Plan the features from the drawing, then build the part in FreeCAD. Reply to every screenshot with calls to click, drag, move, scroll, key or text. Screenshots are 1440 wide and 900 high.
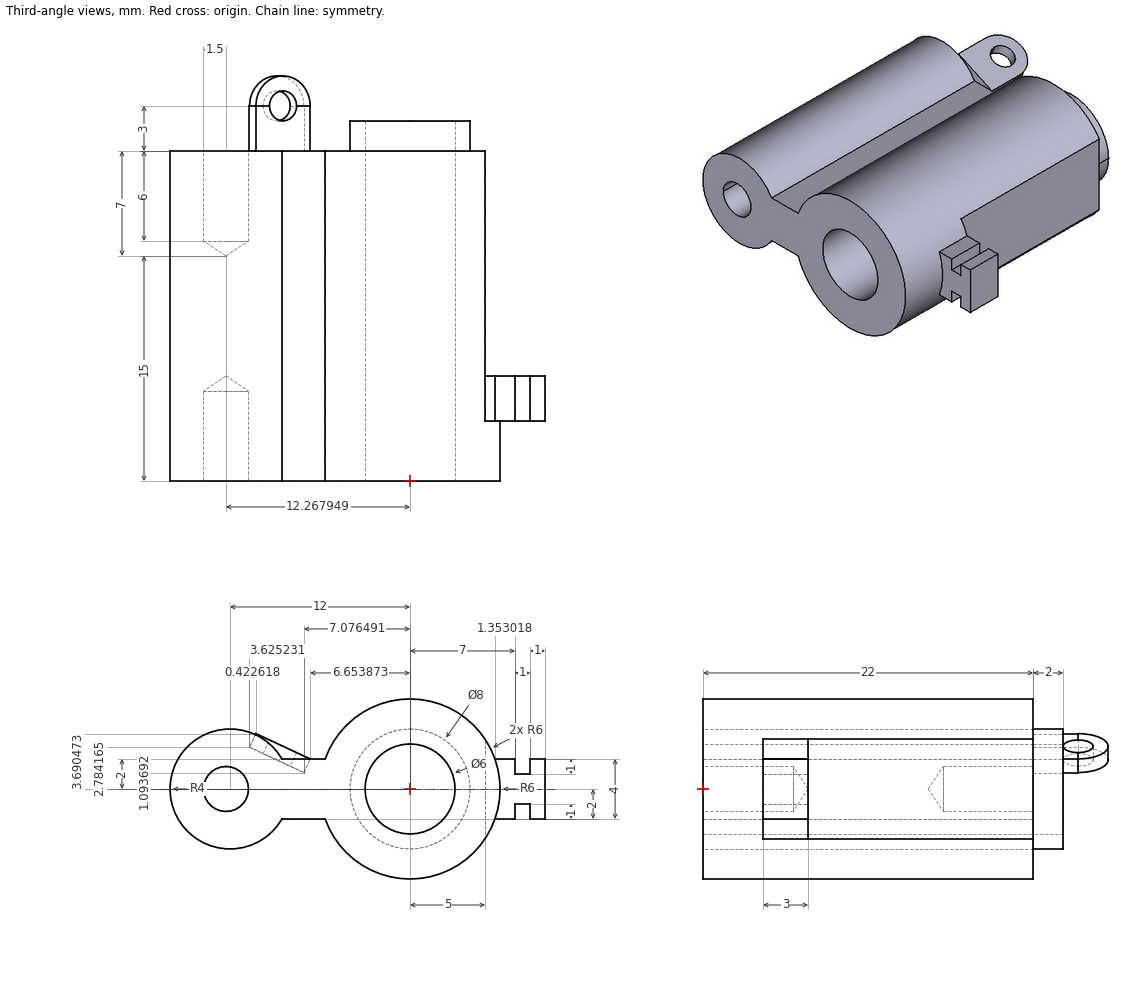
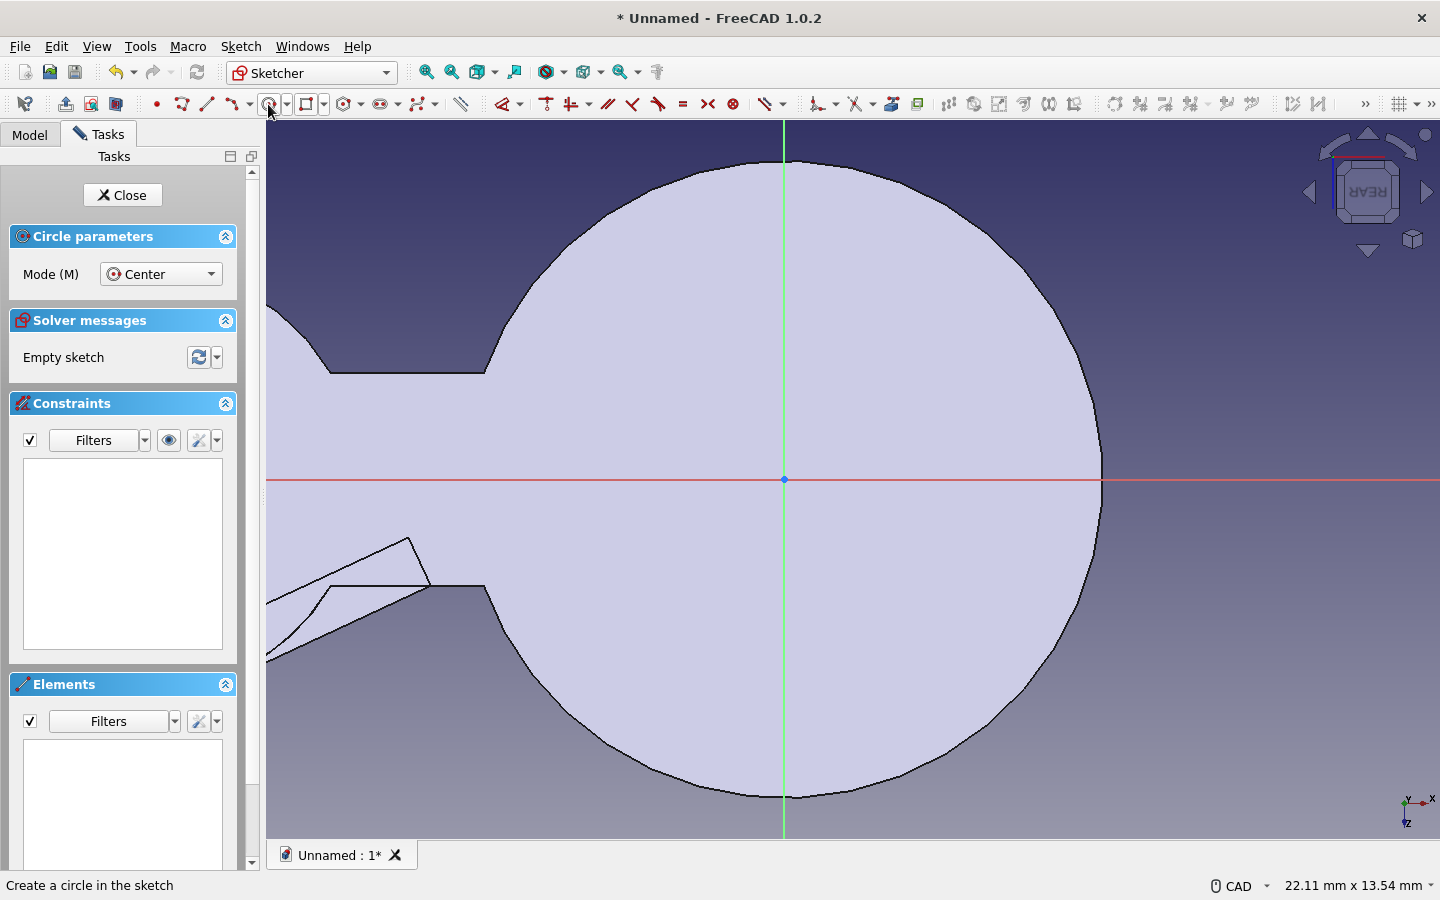
click(784, 479)
move(934, 329)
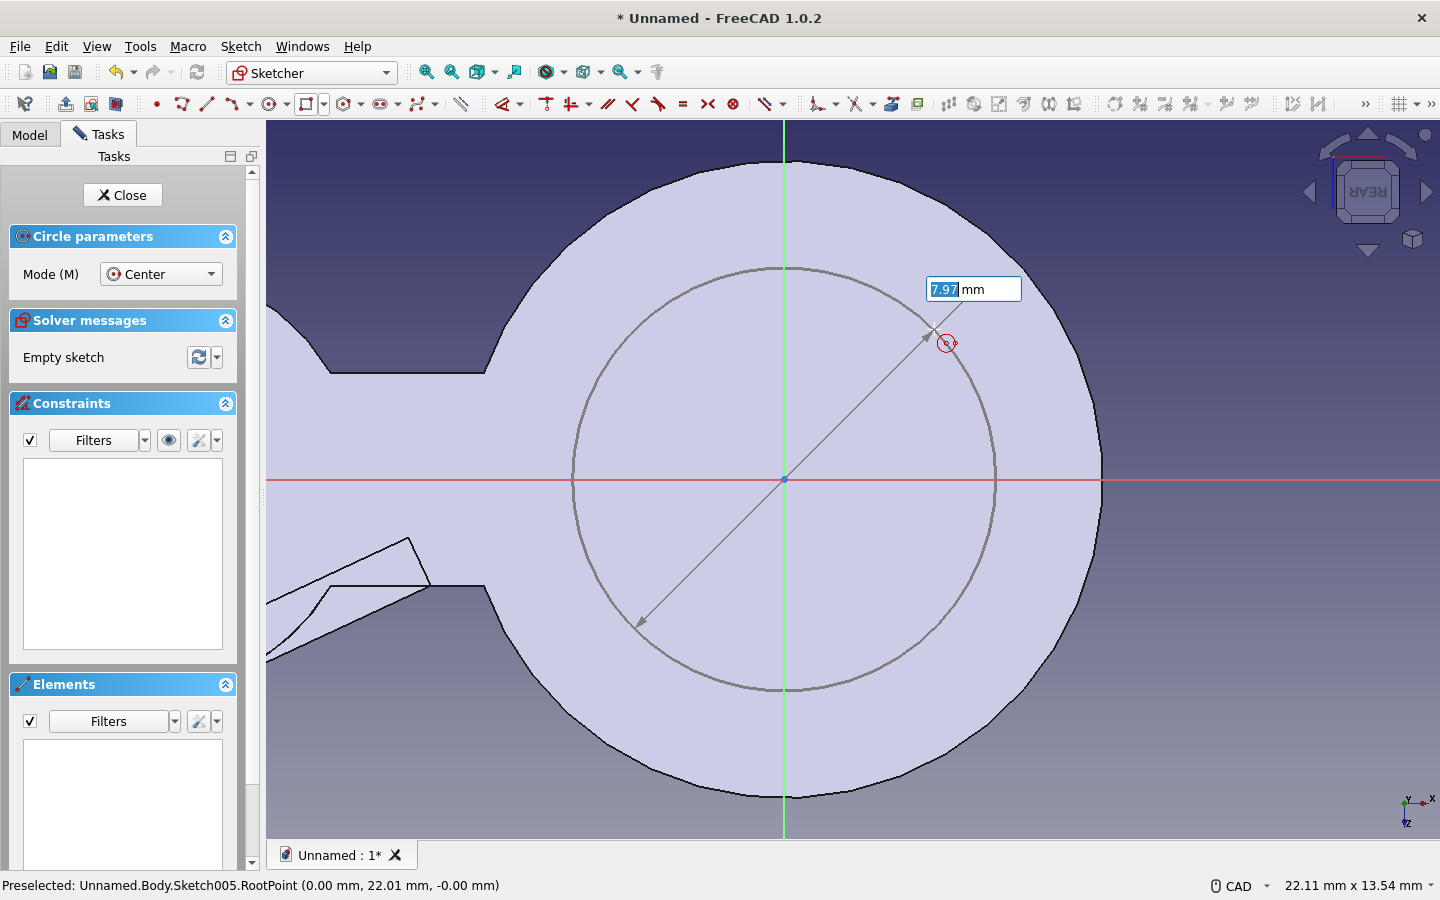
text(8)
key(Return)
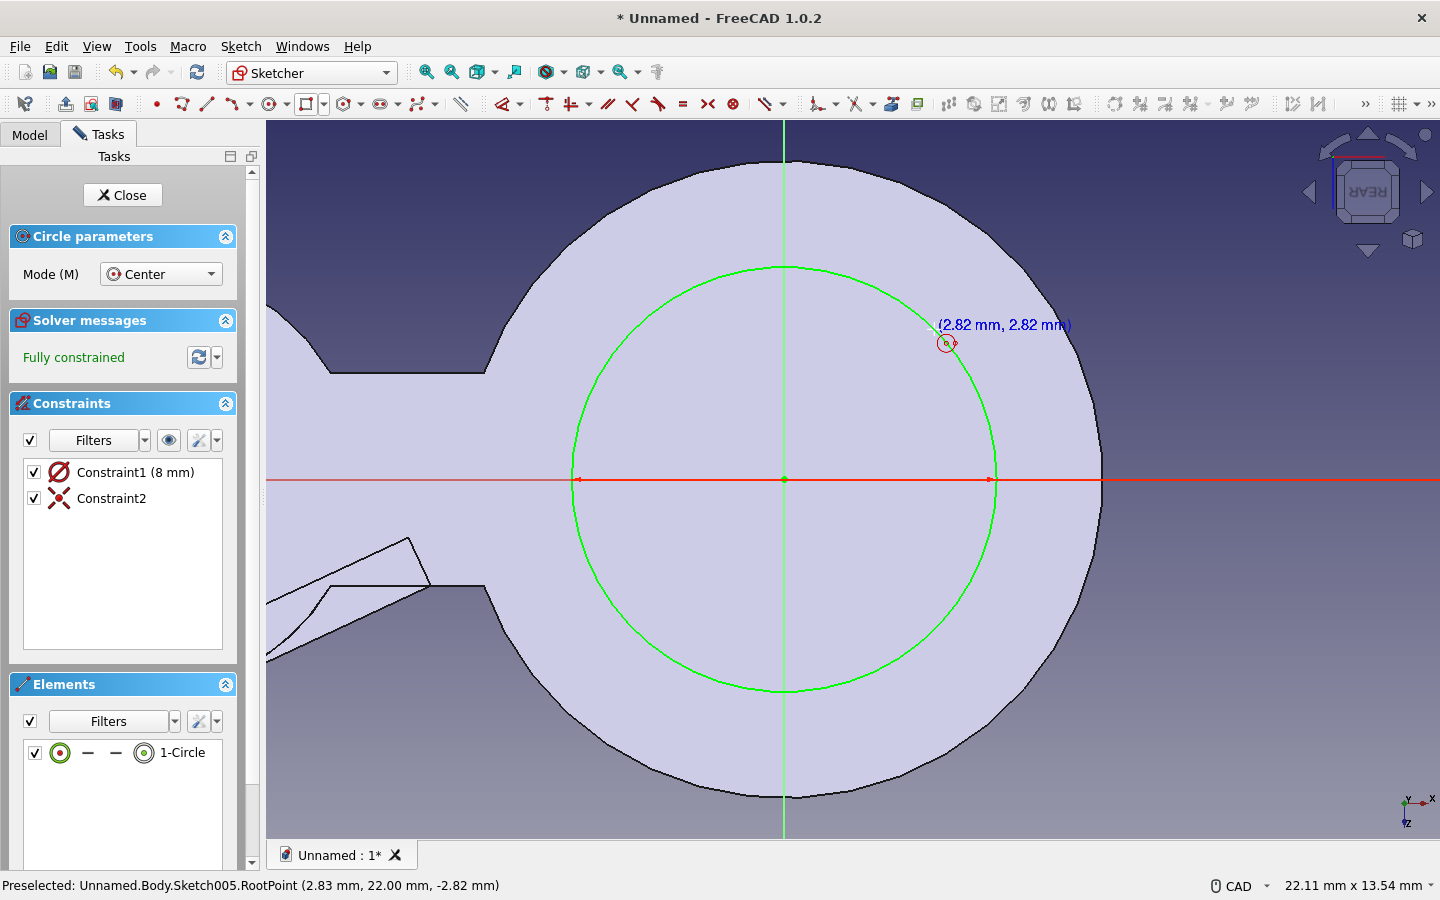
click(784, 479)
move(897, 367)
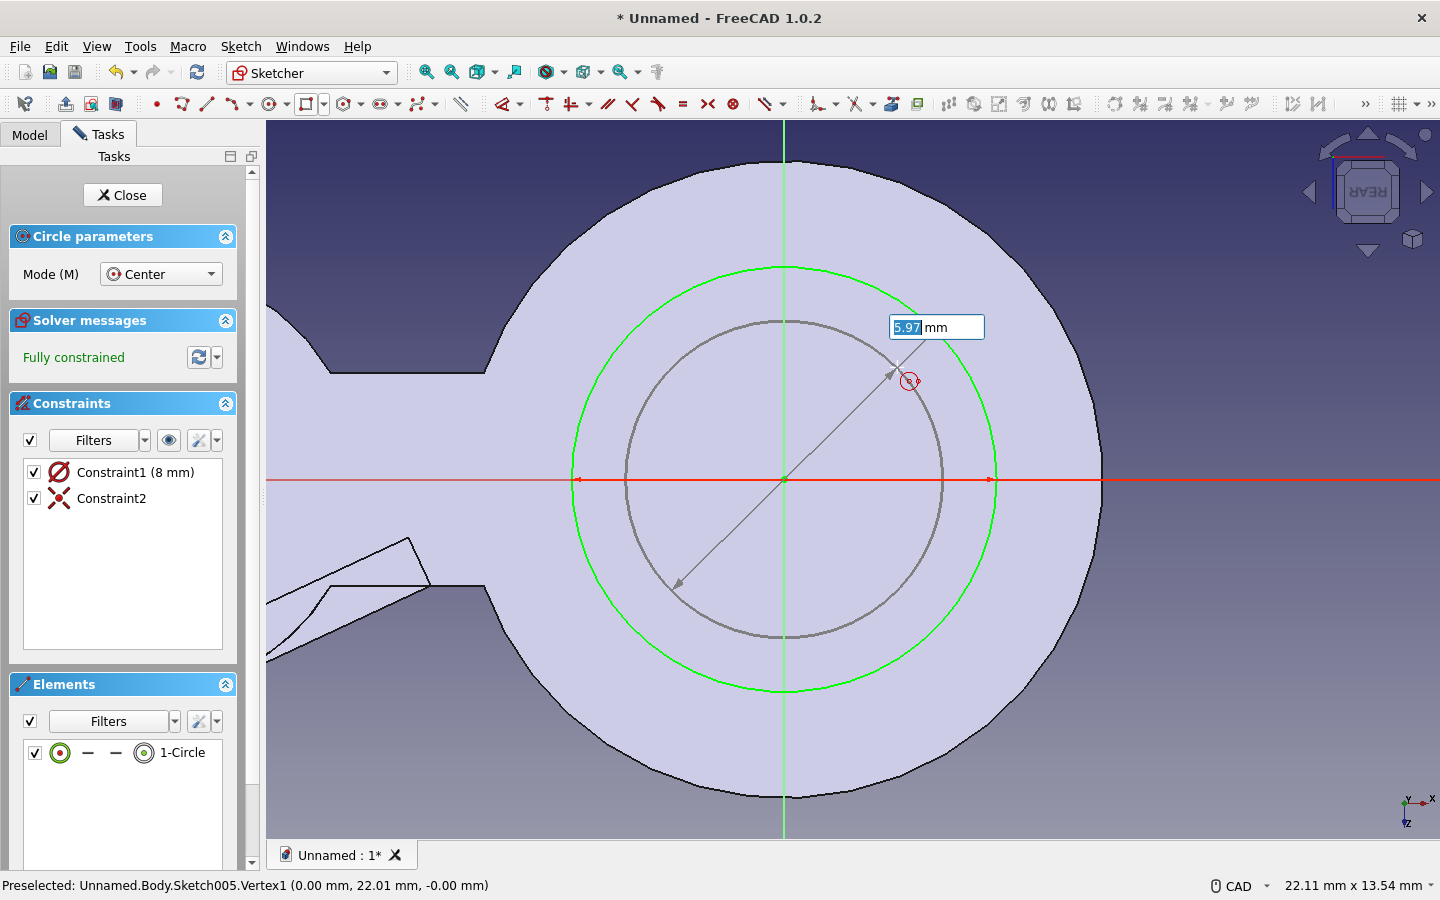
text(6)
key(Return)
key(Escape)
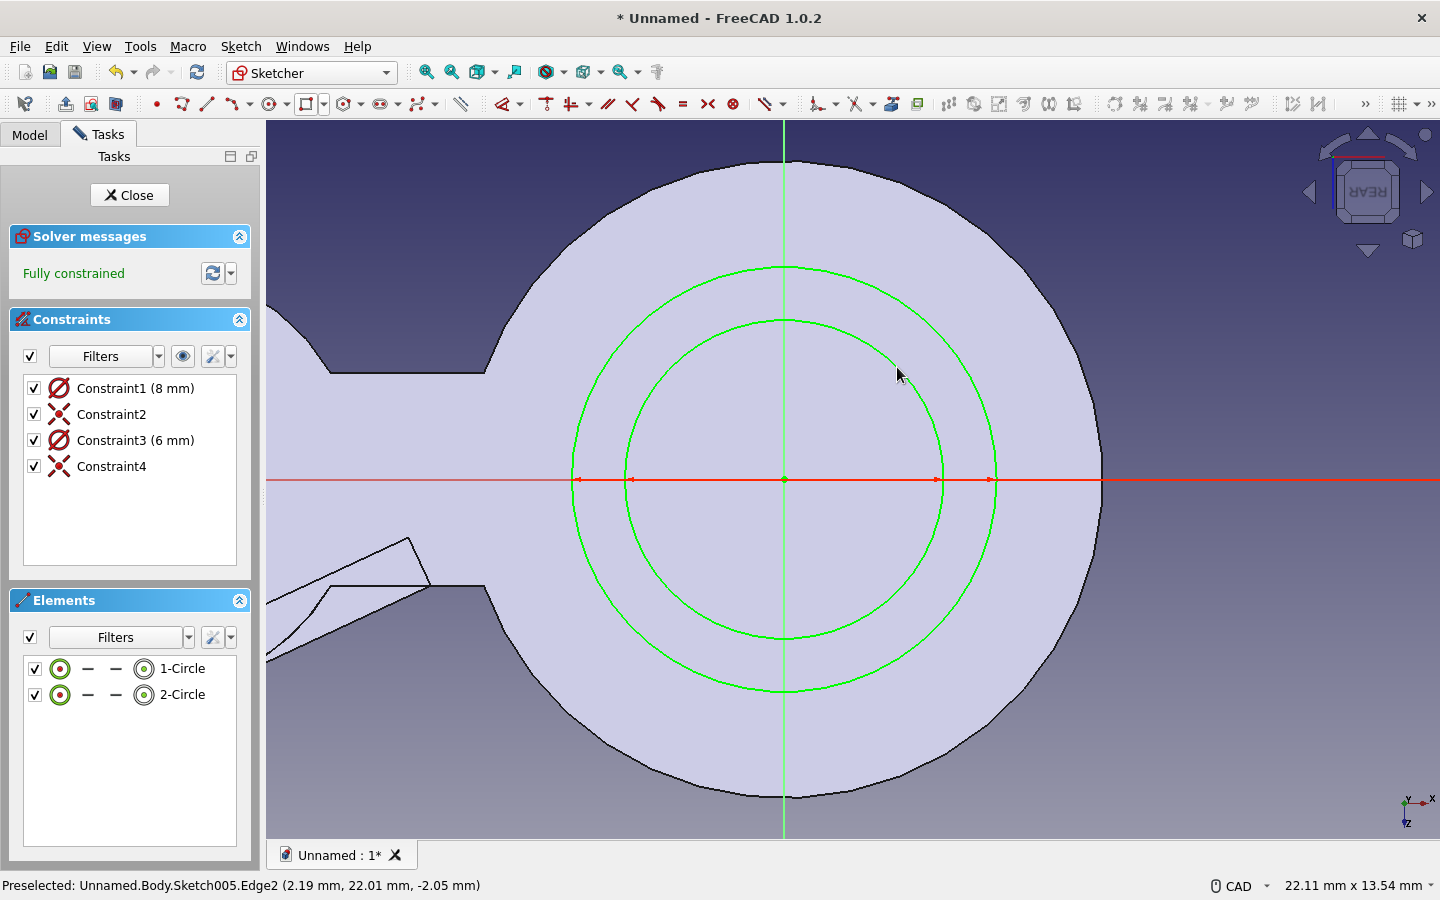
click(130, 195)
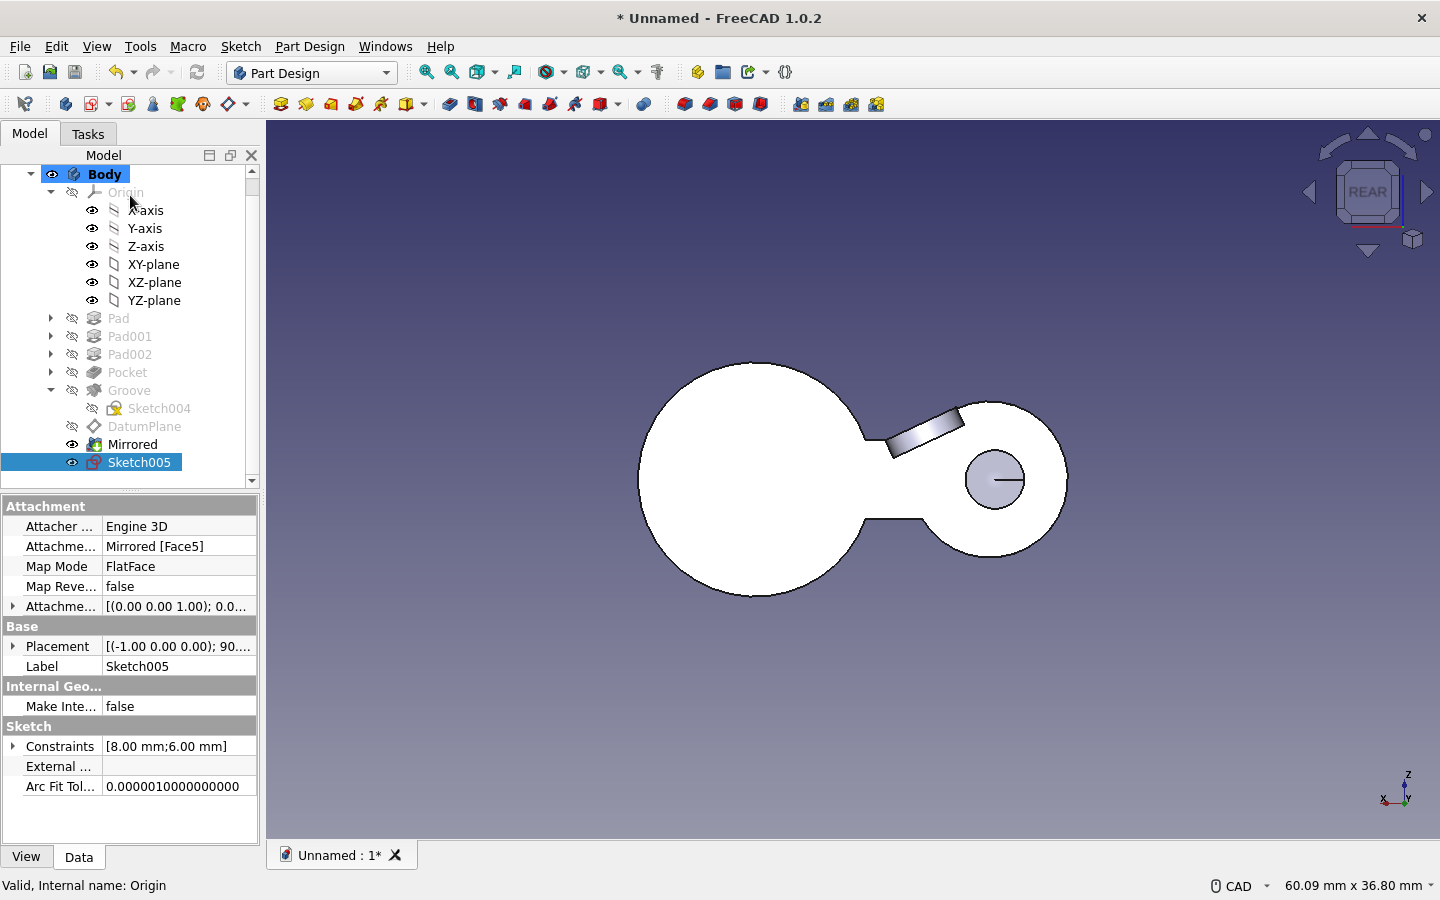
click(281, 104)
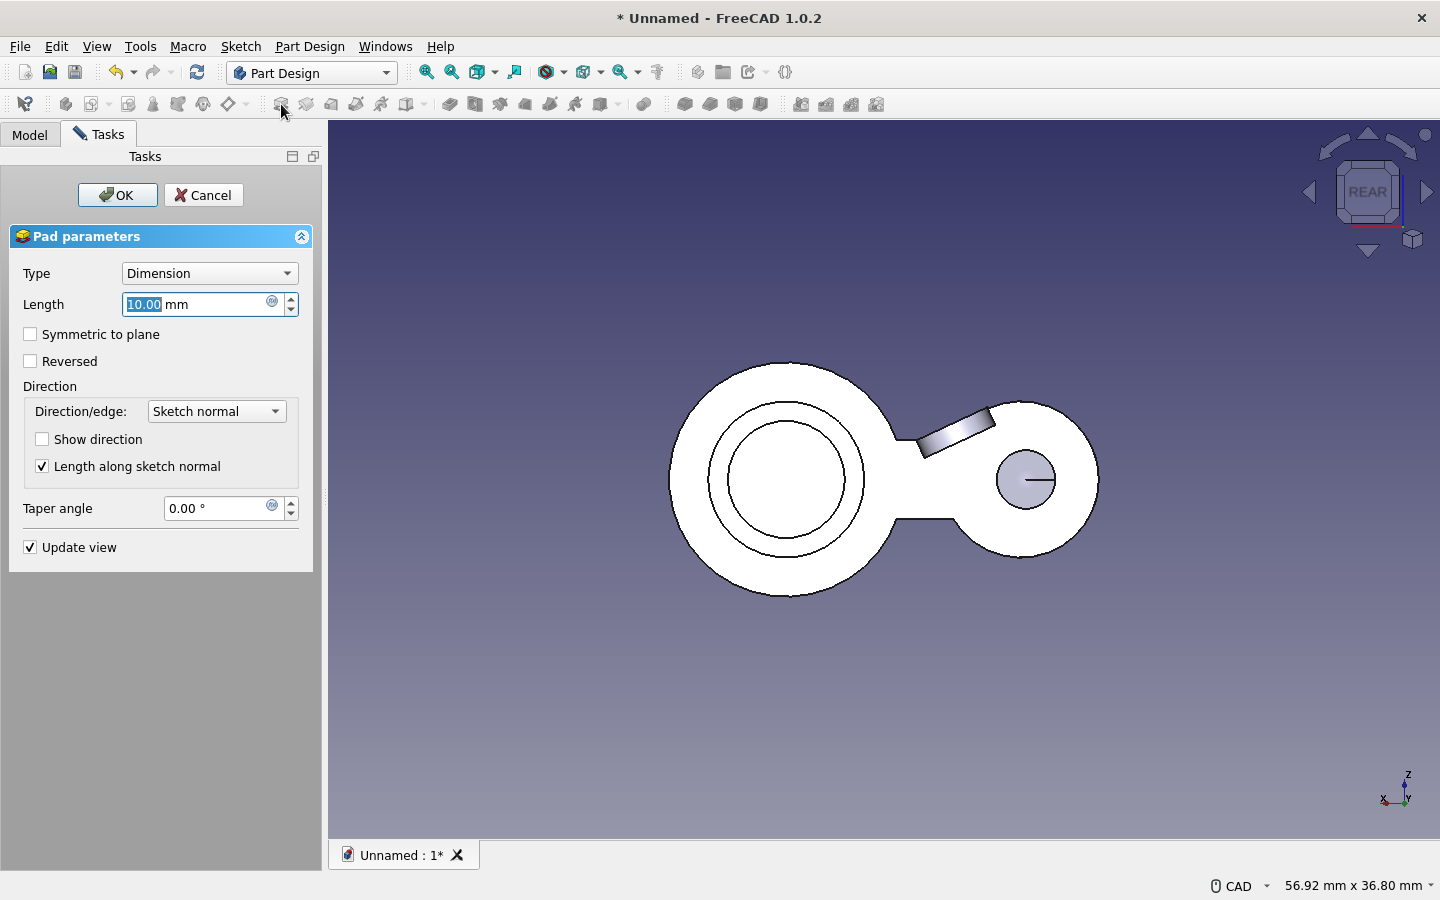
text(2)
key(Tab)